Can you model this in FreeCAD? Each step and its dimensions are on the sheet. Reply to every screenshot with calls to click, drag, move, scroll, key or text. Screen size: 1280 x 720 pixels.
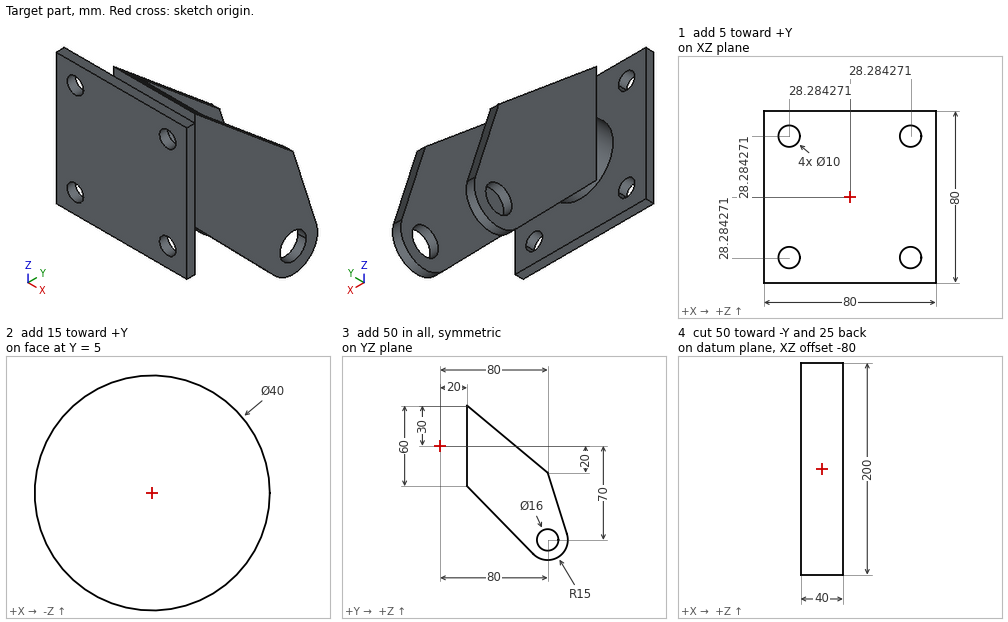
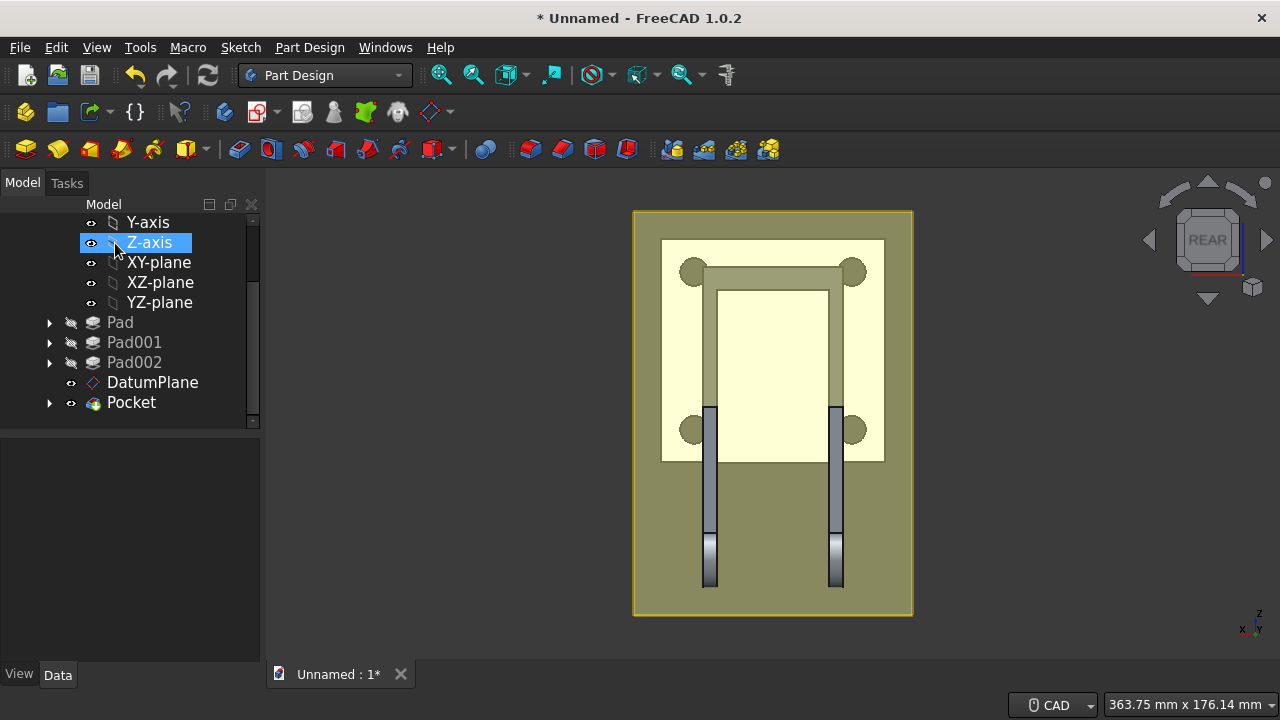
click(116, 383)
key(space)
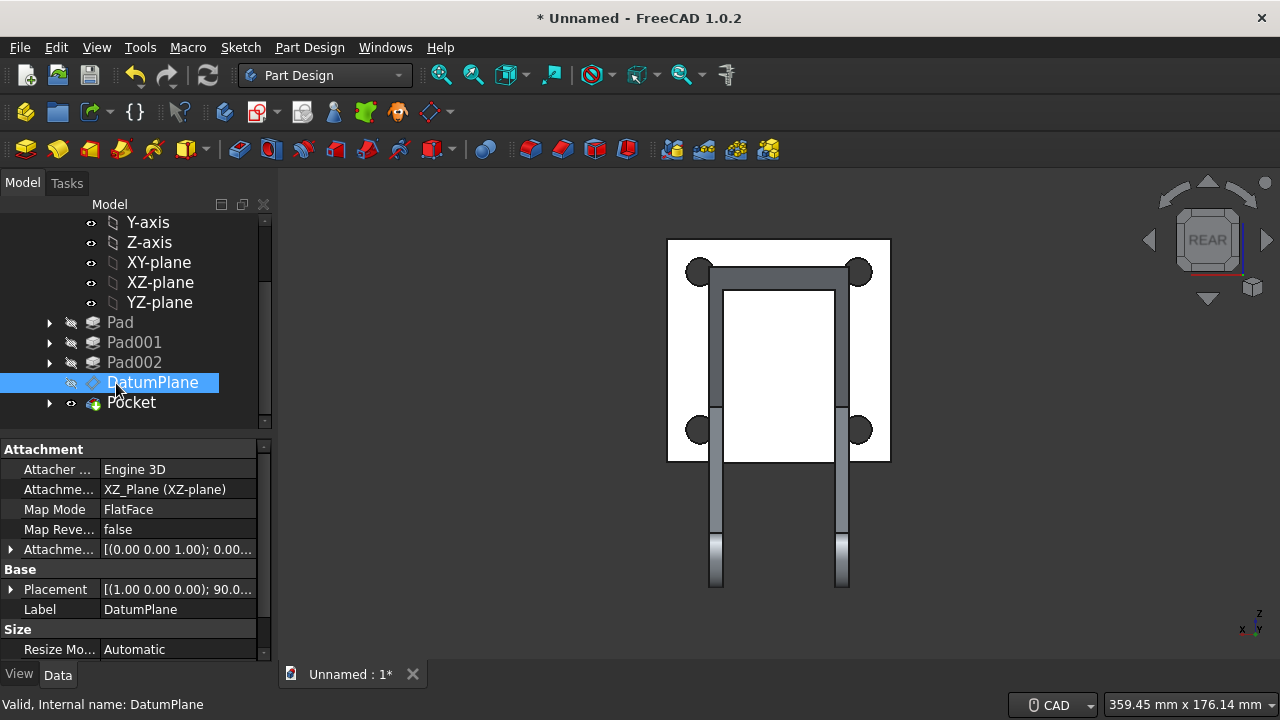
key(0)